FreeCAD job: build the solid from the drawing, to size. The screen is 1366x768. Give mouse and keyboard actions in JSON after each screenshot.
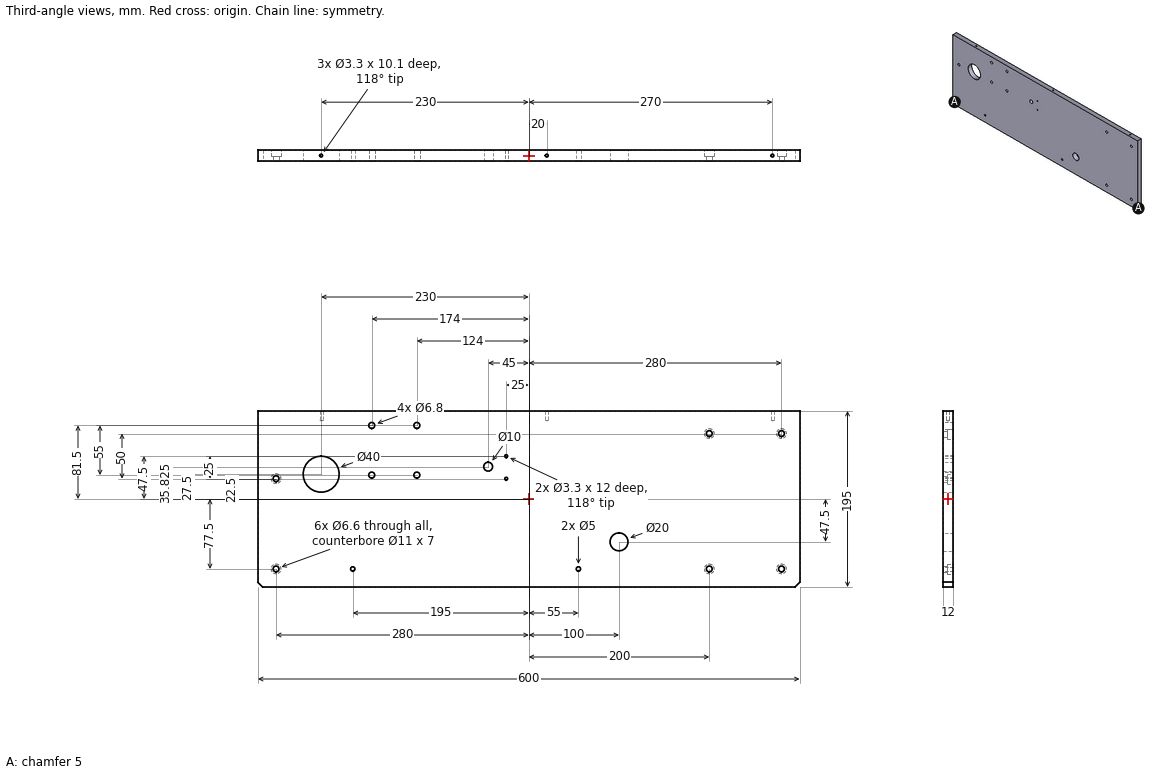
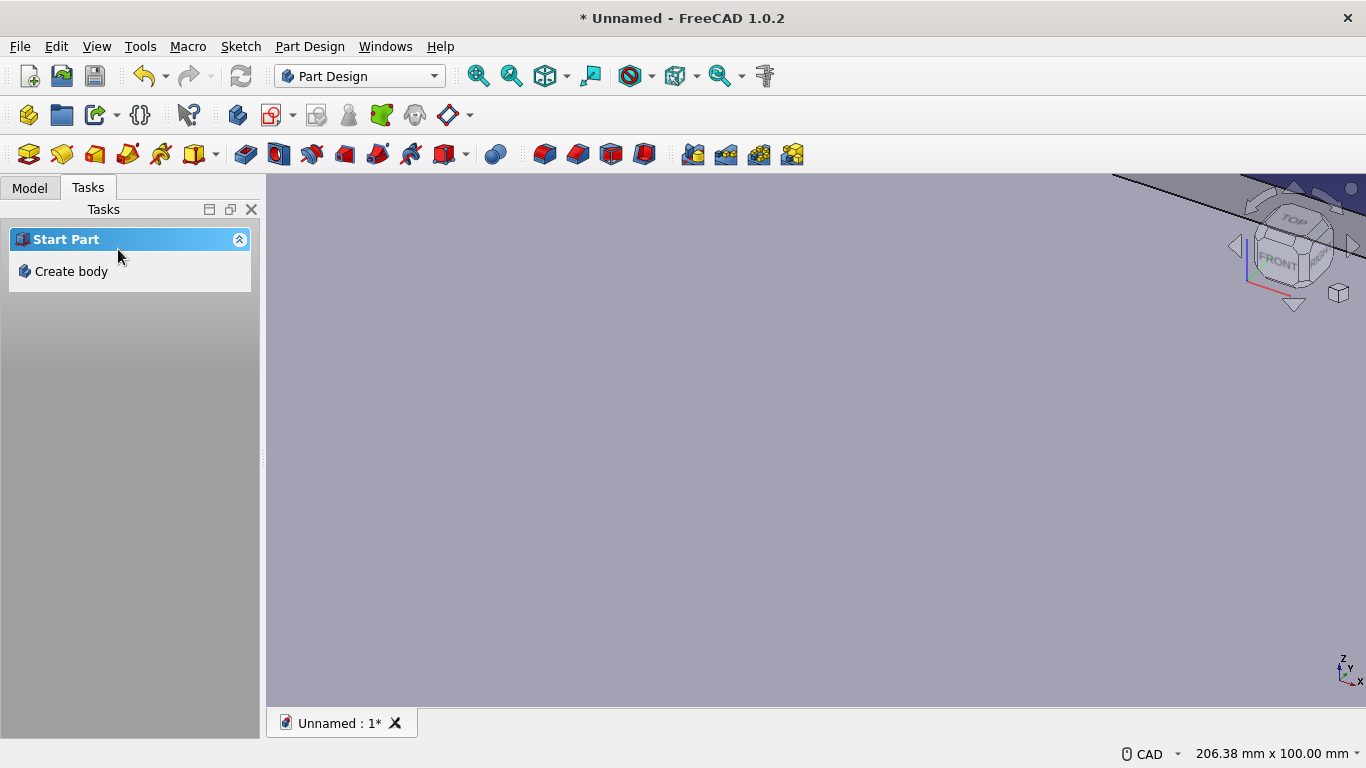
{"action": "key", "text": "v f"}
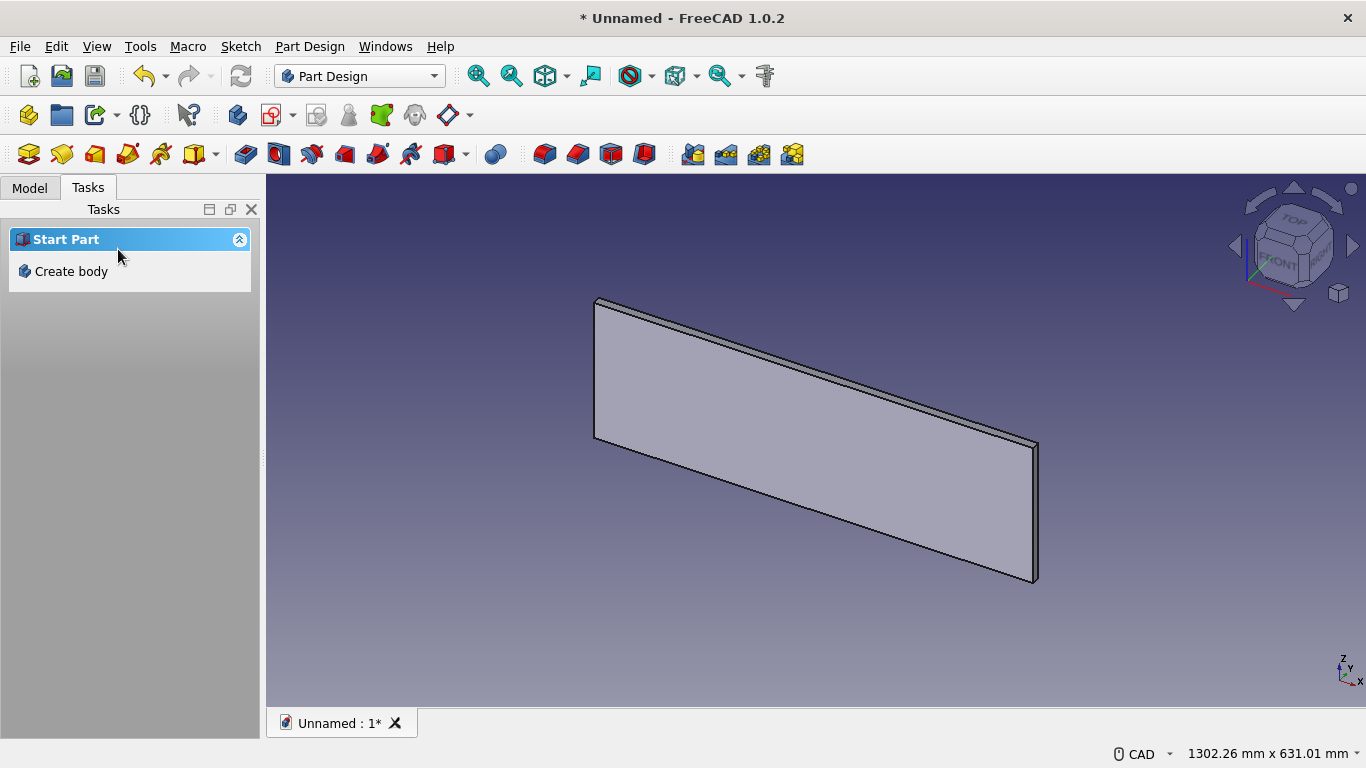
{"action": "scroll", "coordinate": [597, 434], "scroll_direction": "up", "scroll_amount": 7}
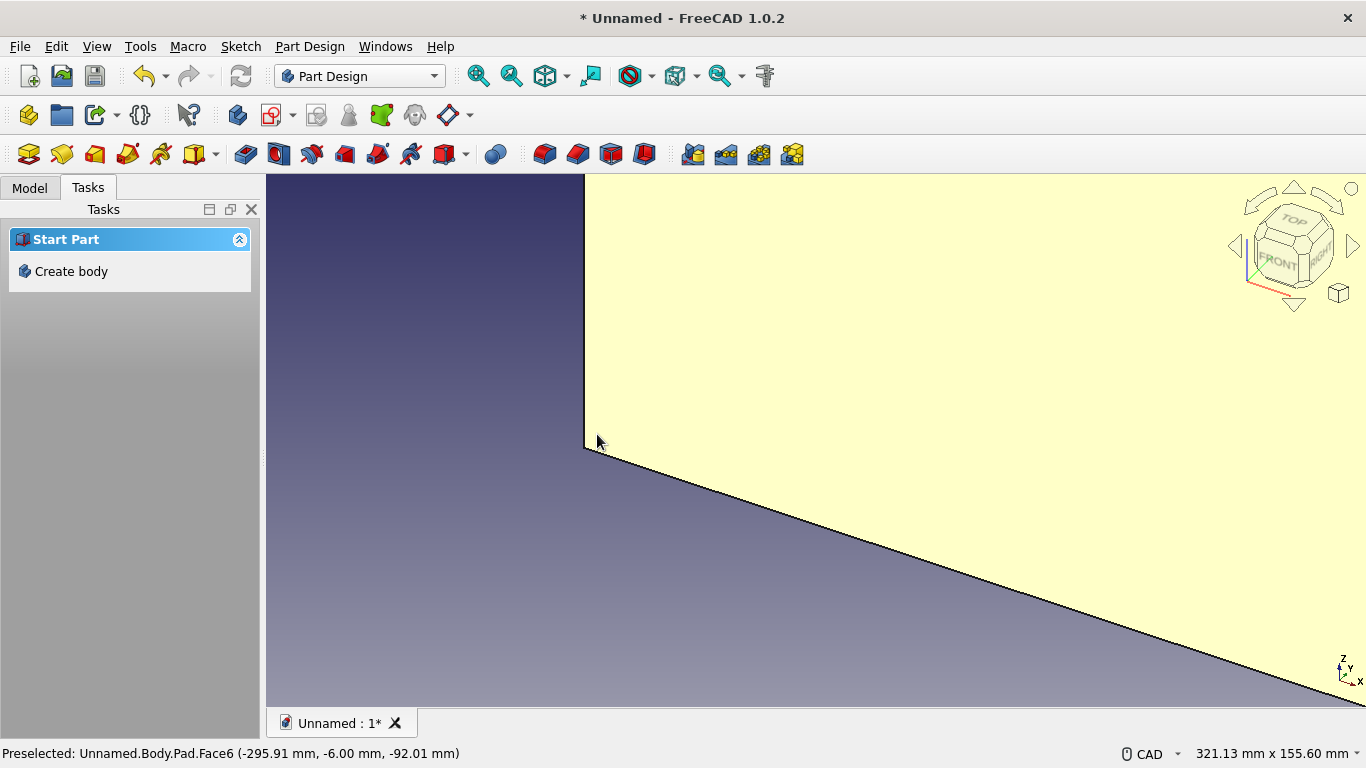
{"action": "key", "text": "v f"}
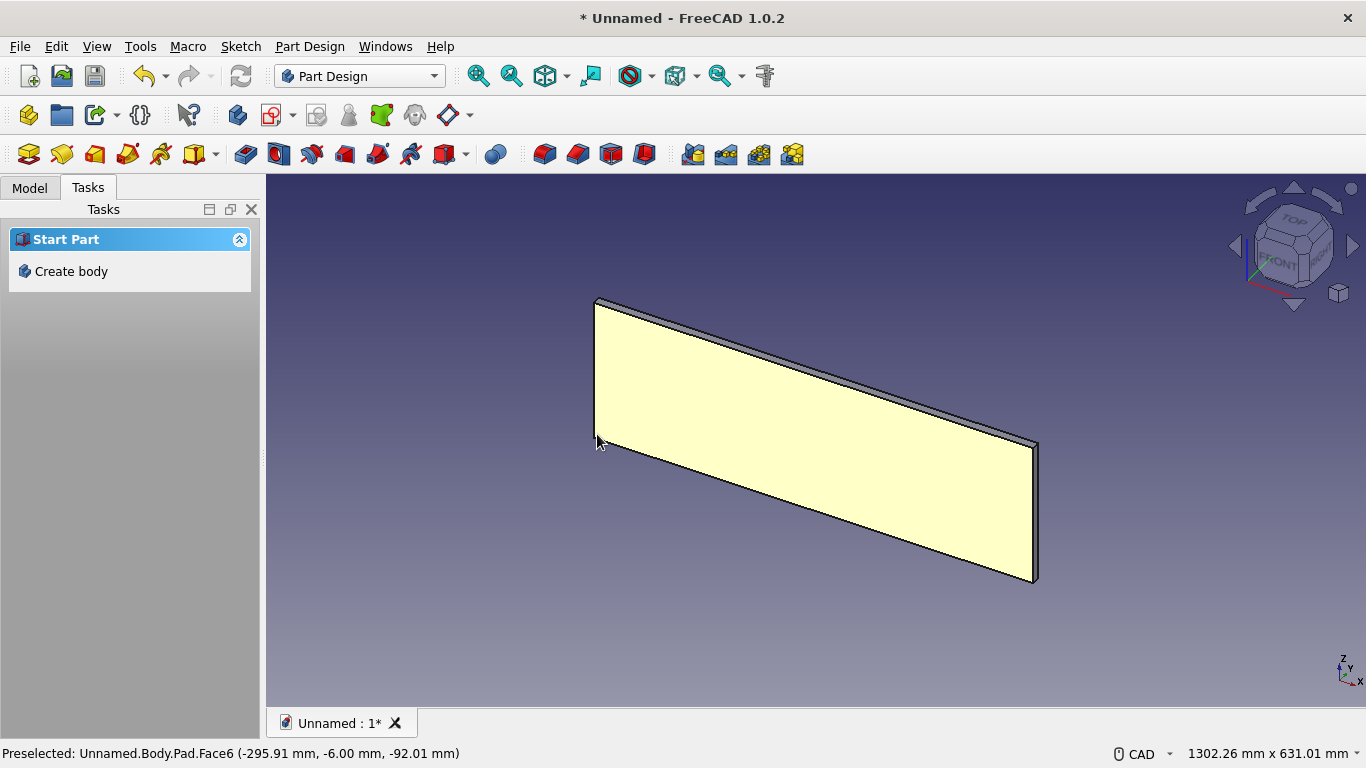
{"action": "key", "text": "0"}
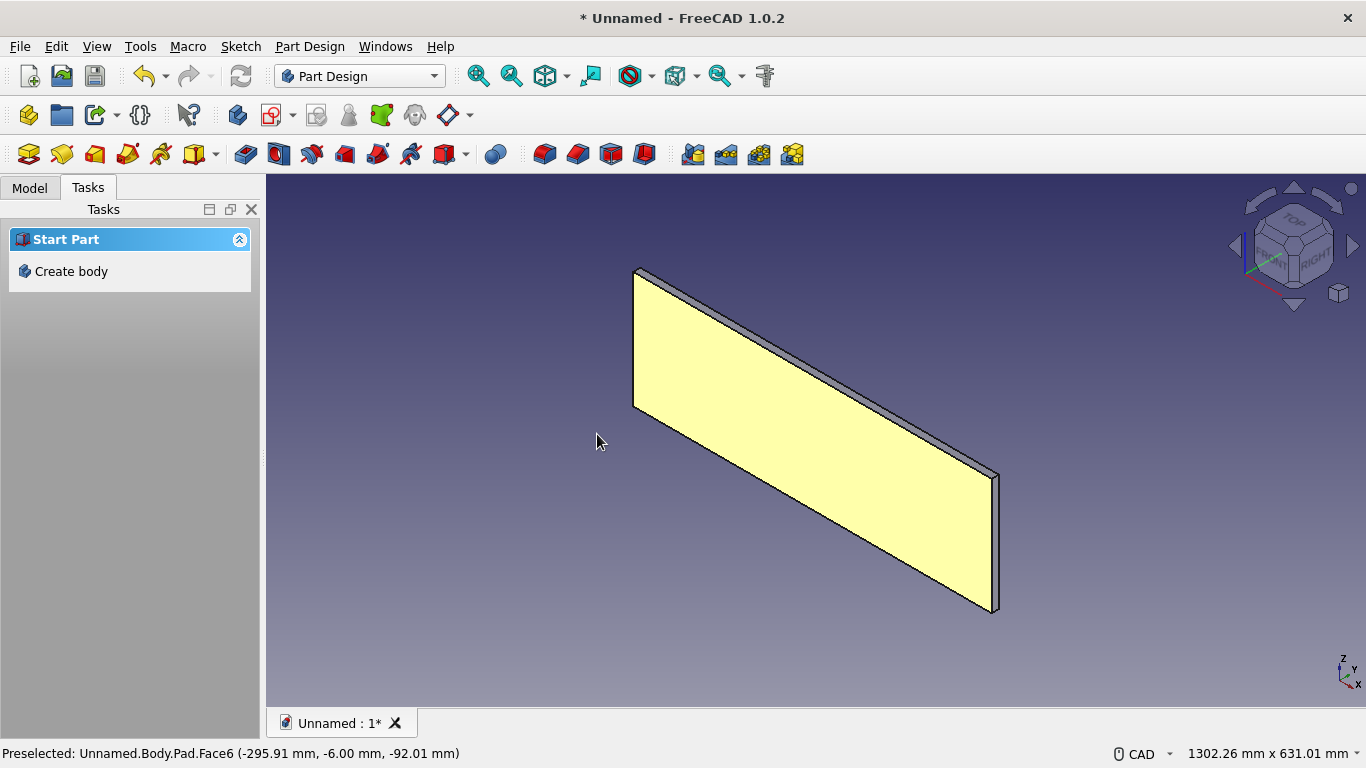
{"action": "scroll", "coordinate": [637, 403], "scroll_direction": "up", "scroll_amount": 7}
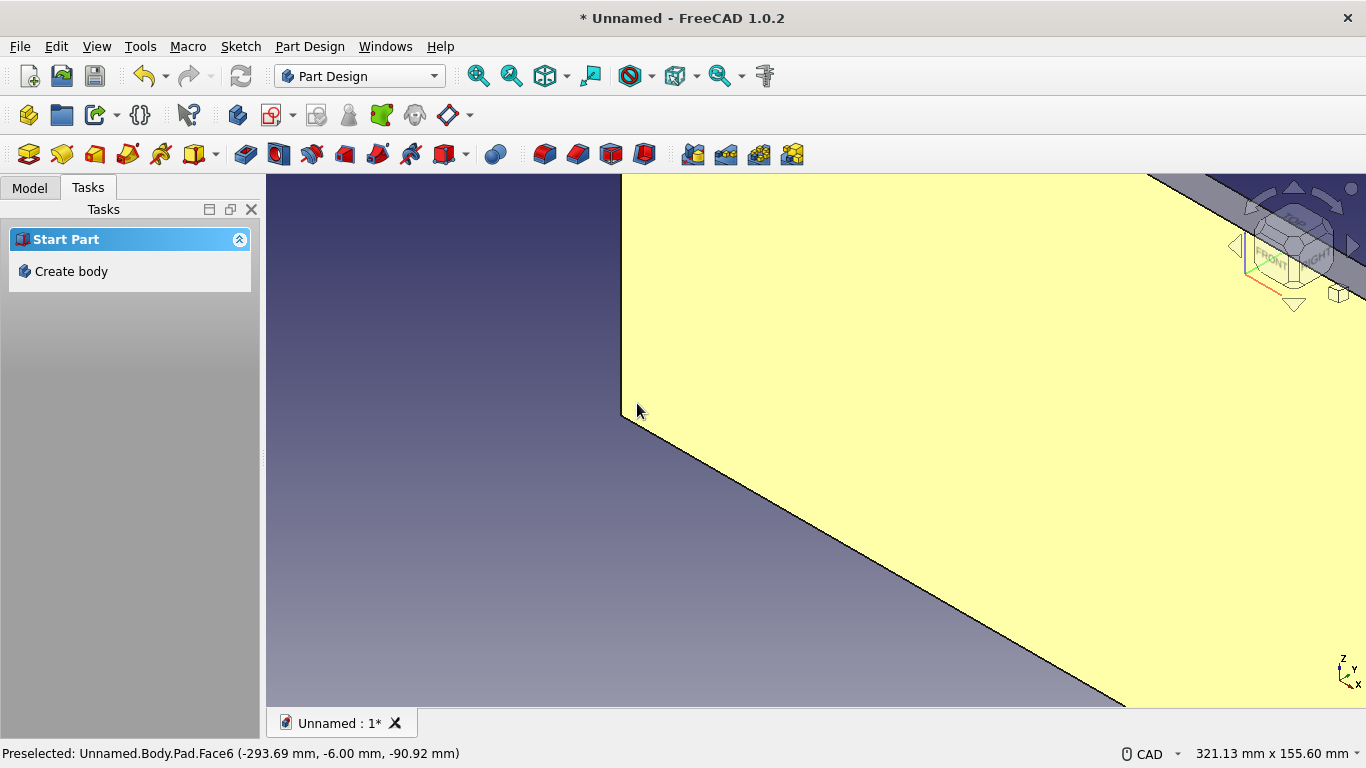
{"action": "key", "text": "v f"}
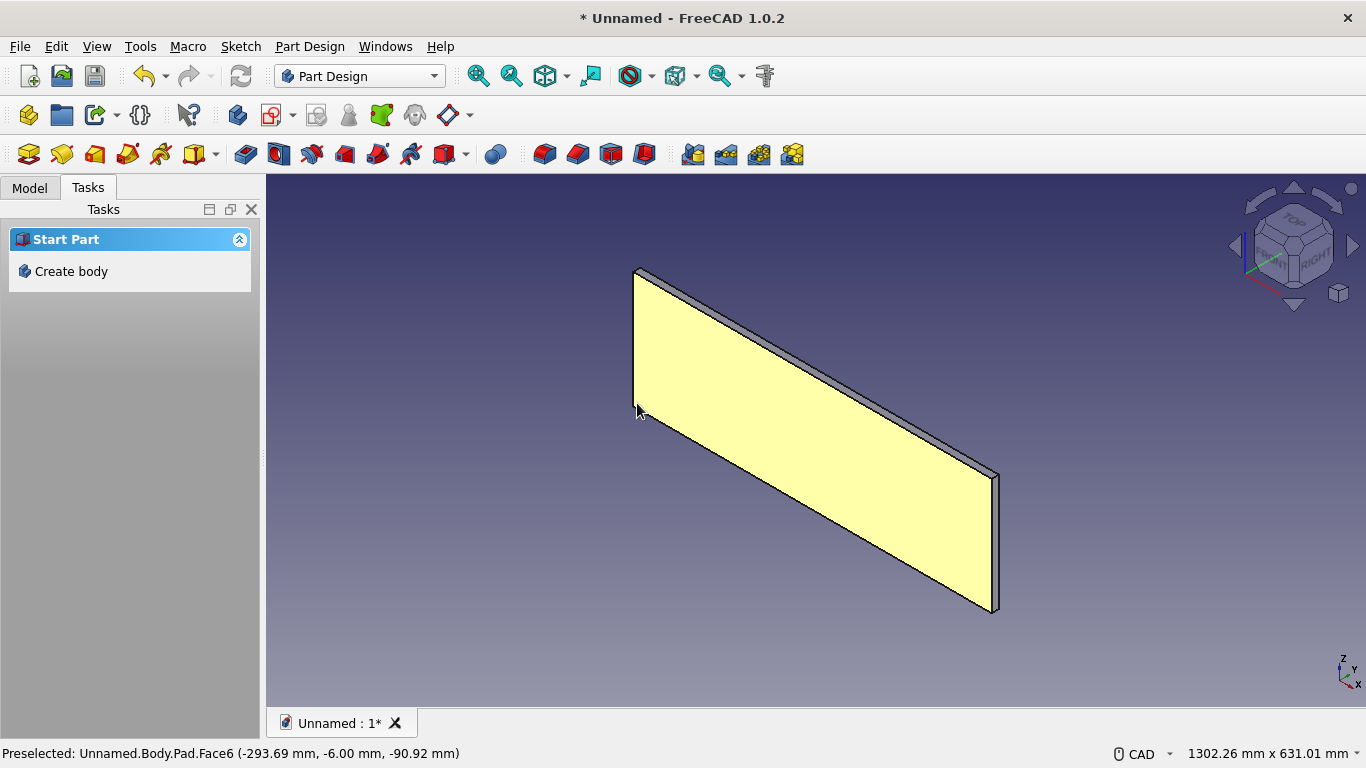
{"action": "key", "text": "2"}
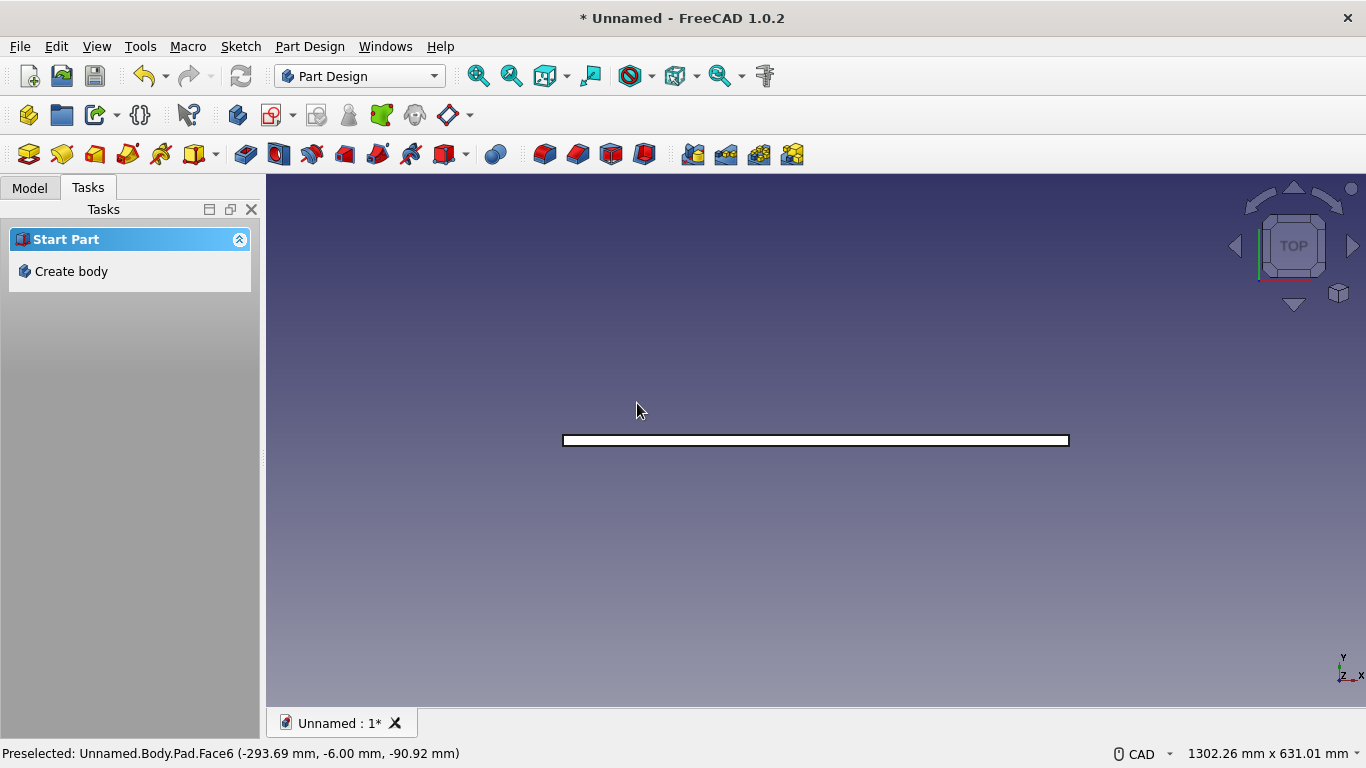
{"action": "scroll", "coordinate": [563, 439], "scroll_direction": "up", "scroll_amount": 7}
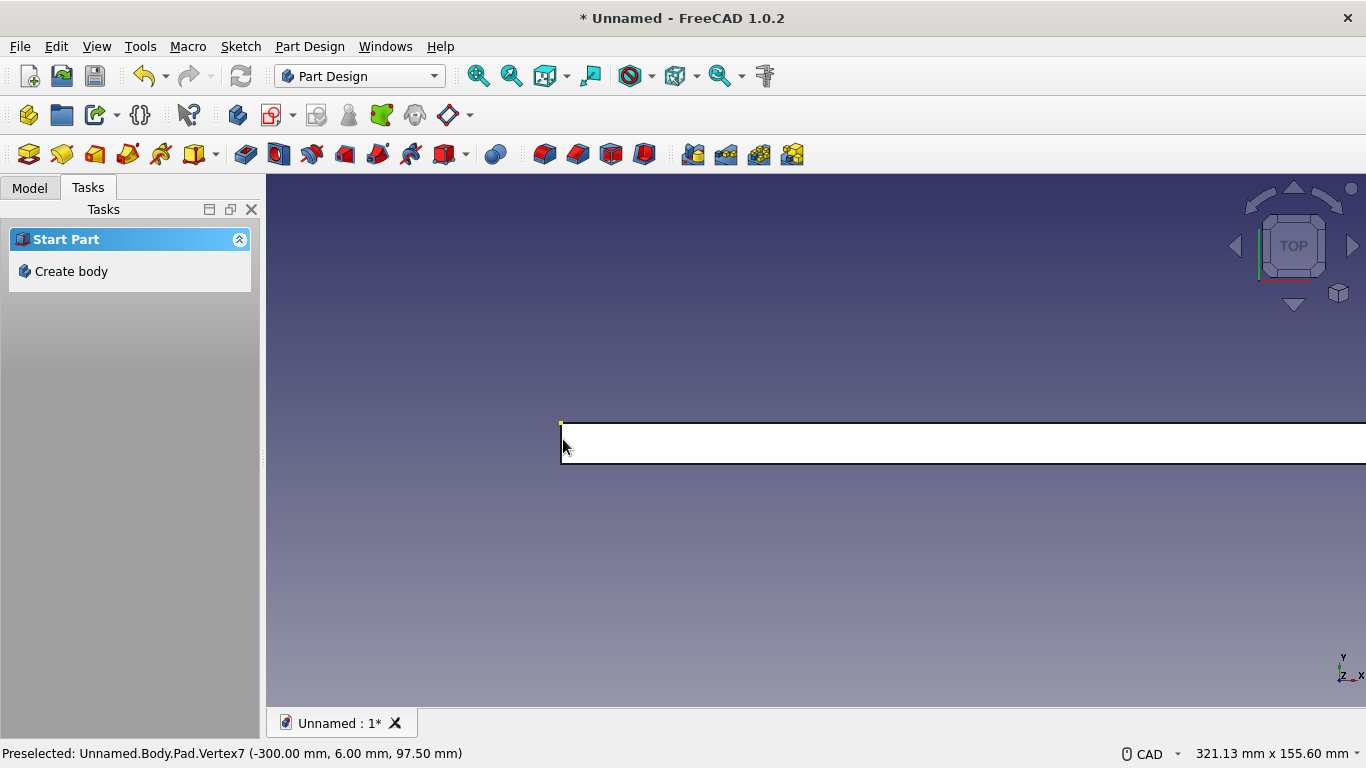
{"action": "key", "text": "v f"}